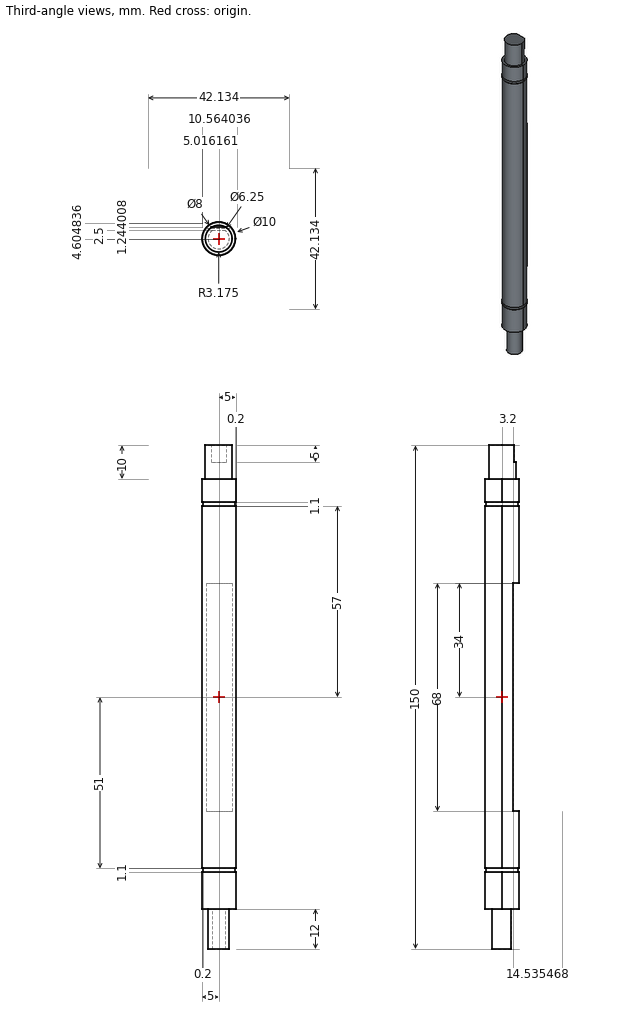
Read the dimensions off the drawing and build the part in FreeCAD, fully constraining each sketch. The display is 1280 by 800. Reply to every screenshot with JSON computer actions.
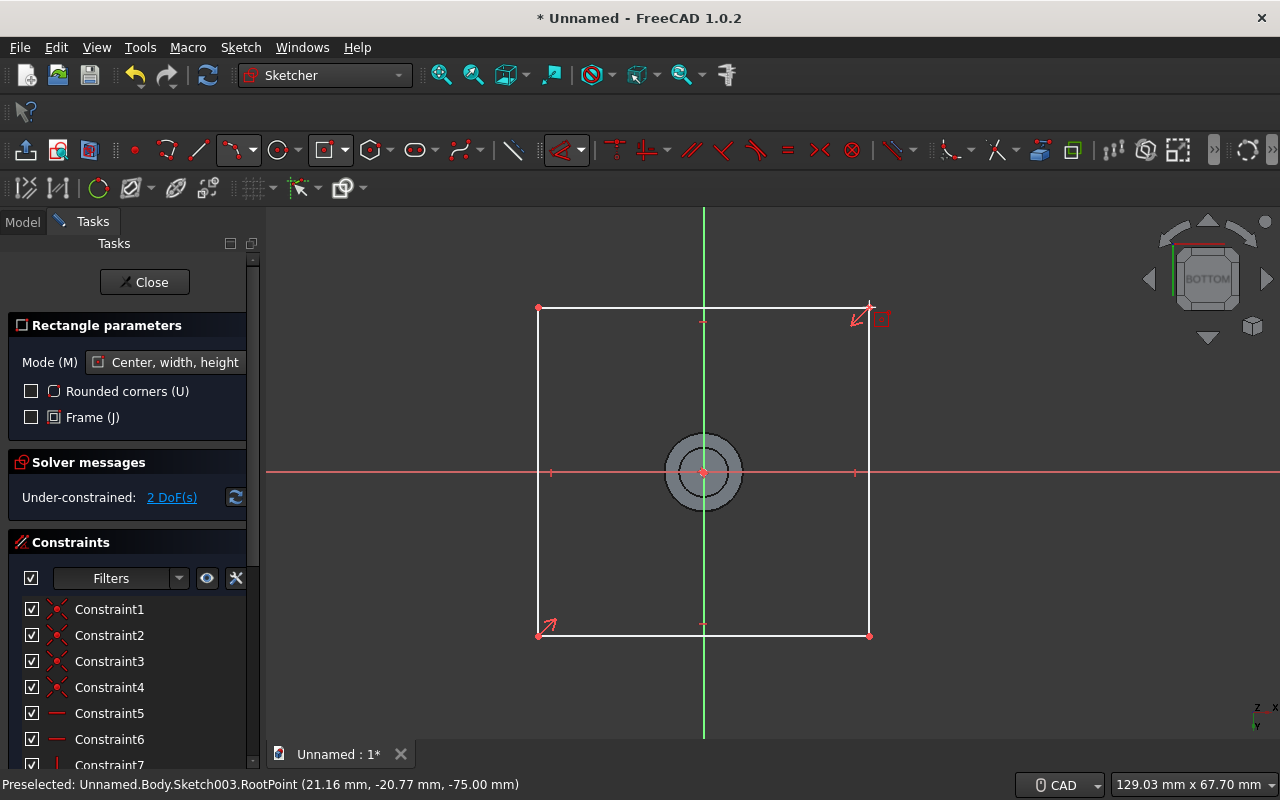
{"action": "left_click", "coordinate": [200, 150]}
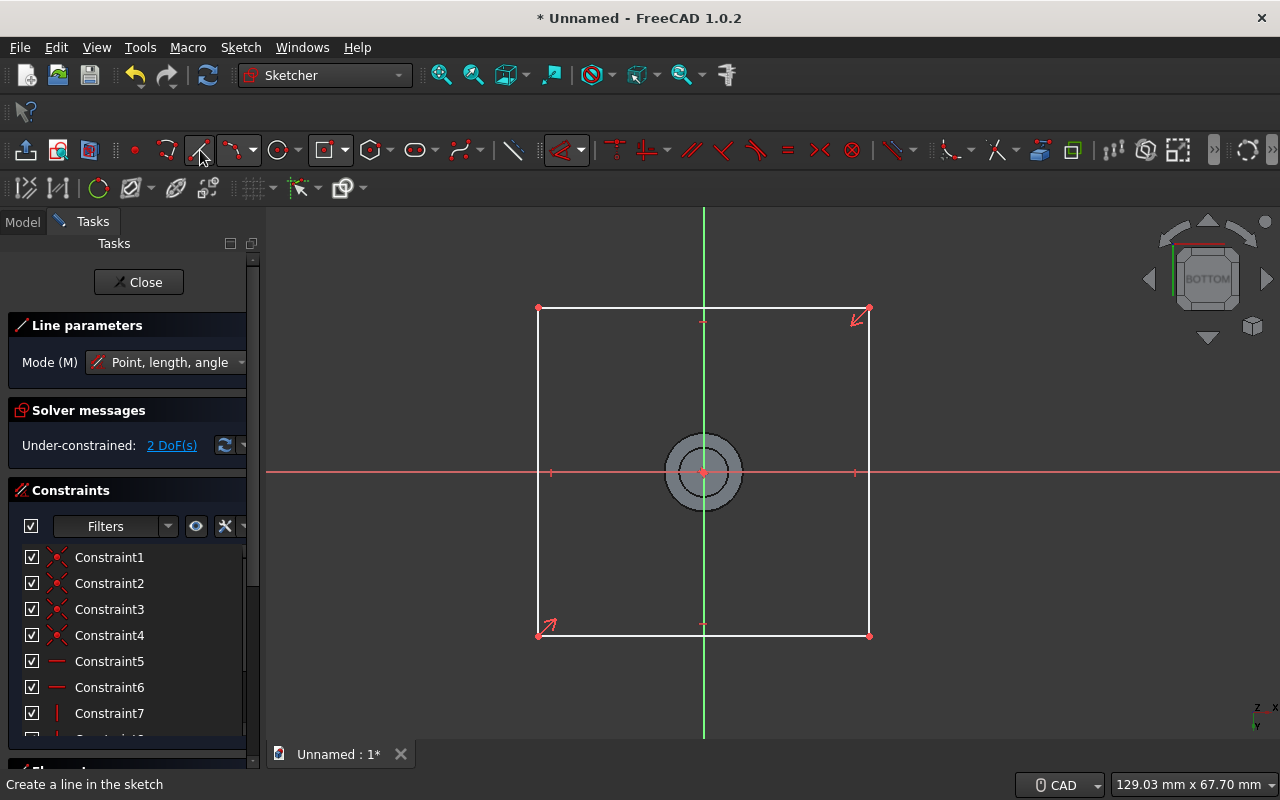
{"action": "left_click", "coordinate": [688, 492]}
{"action": "left_click", "coordinate": [719, 492]}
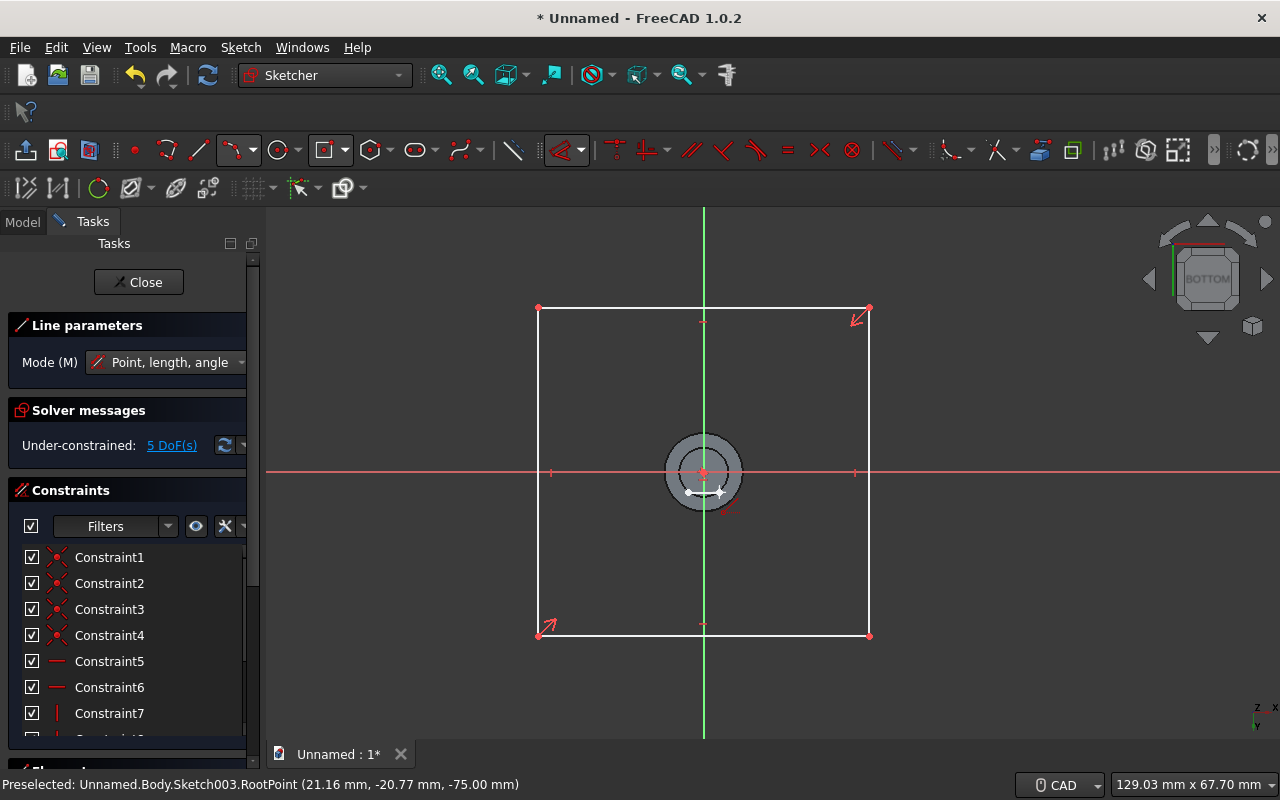
{"action": "left_click", "coordinate": [232, 150]}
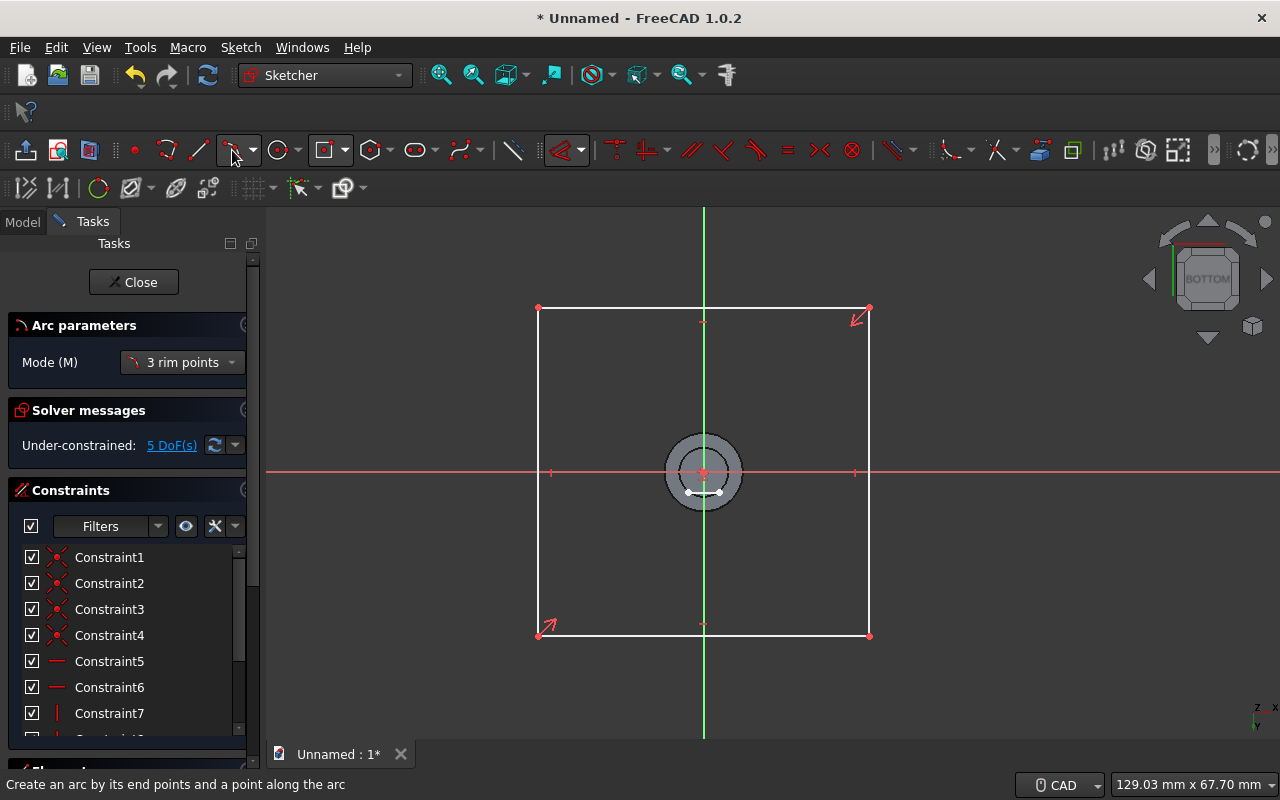
{"action": "left_click", "coordinate": [719, 493]}
{"action": "left_click", "coordinate": [688, 493]}
{"action": "left_click", "coordinate": [683, 459]}
{"action": "key", "text": "Escape"}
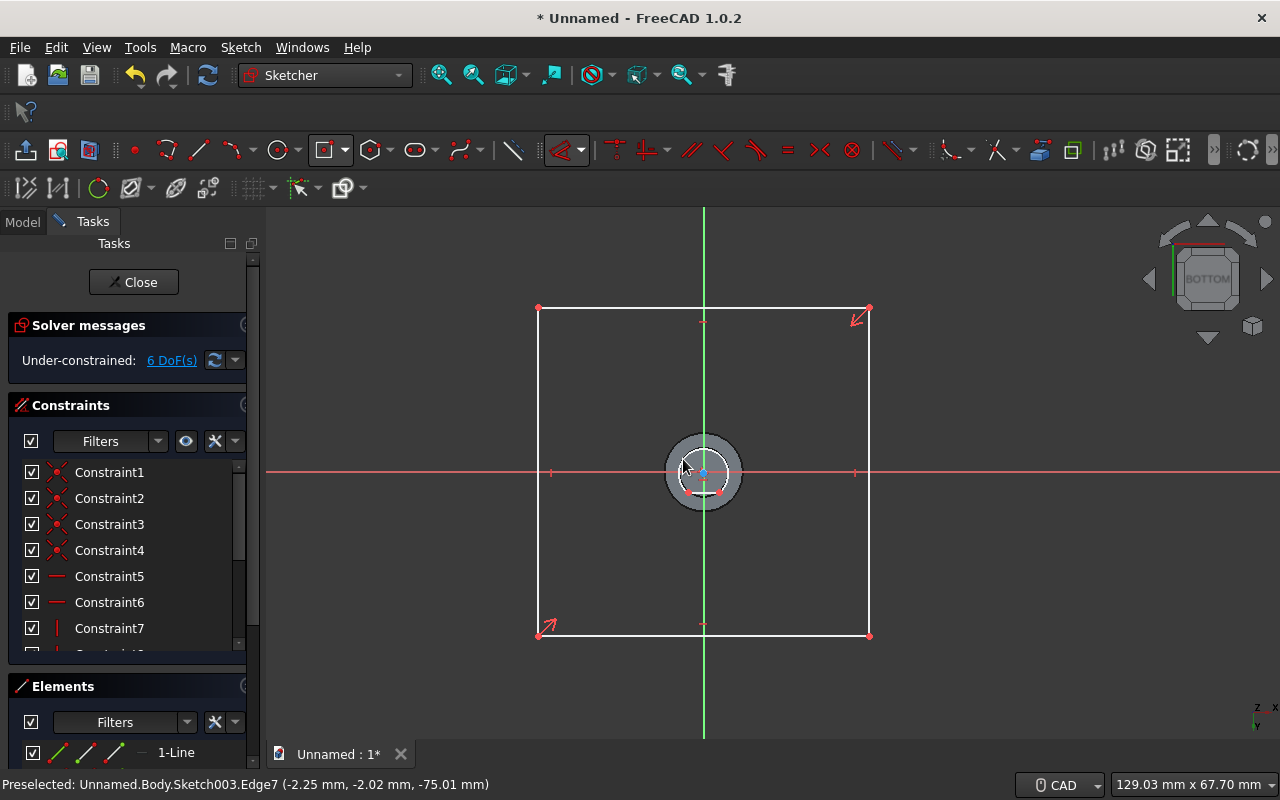
{"action": "scroll", "coordinate": [704, 473], "scroll_direction": "up", "scroll_amount": 3}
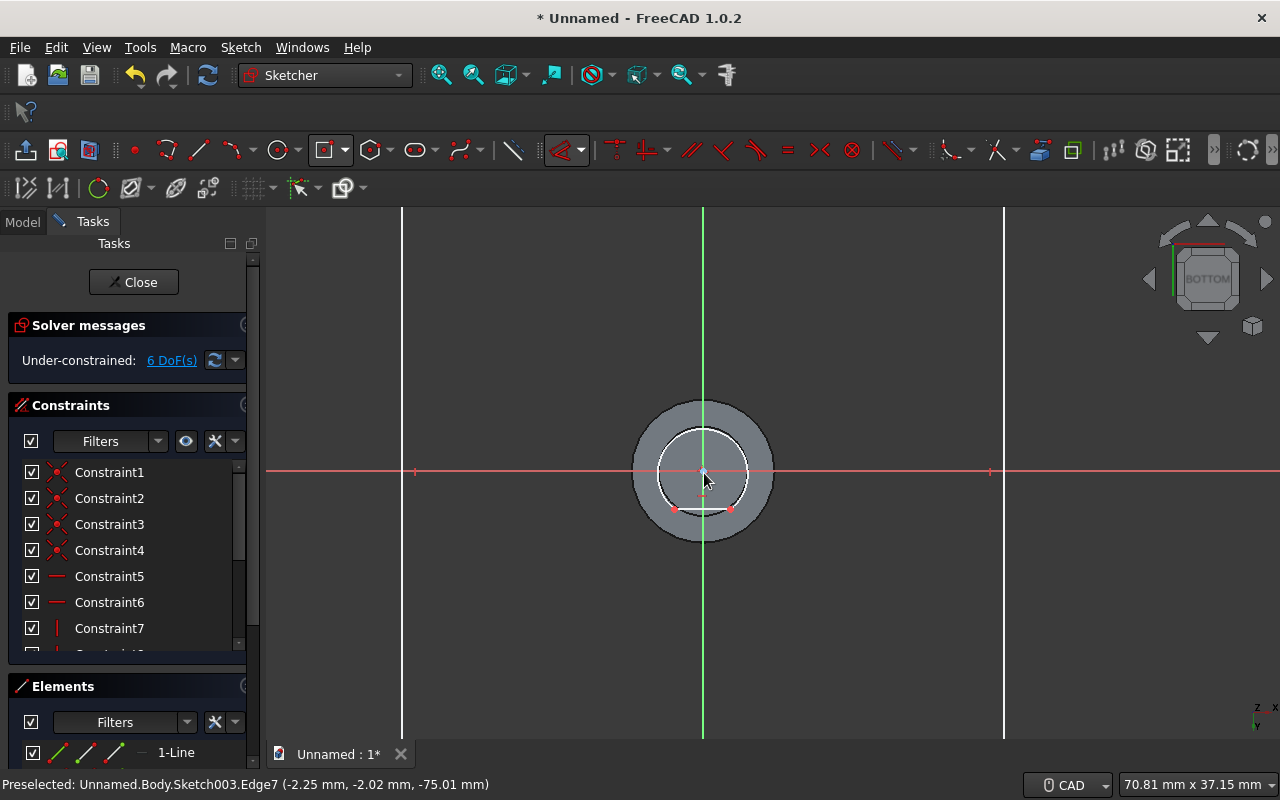
{"action": "left_click_drag", "start_coordinate": [693, 461], "coordinate": [713, 484]}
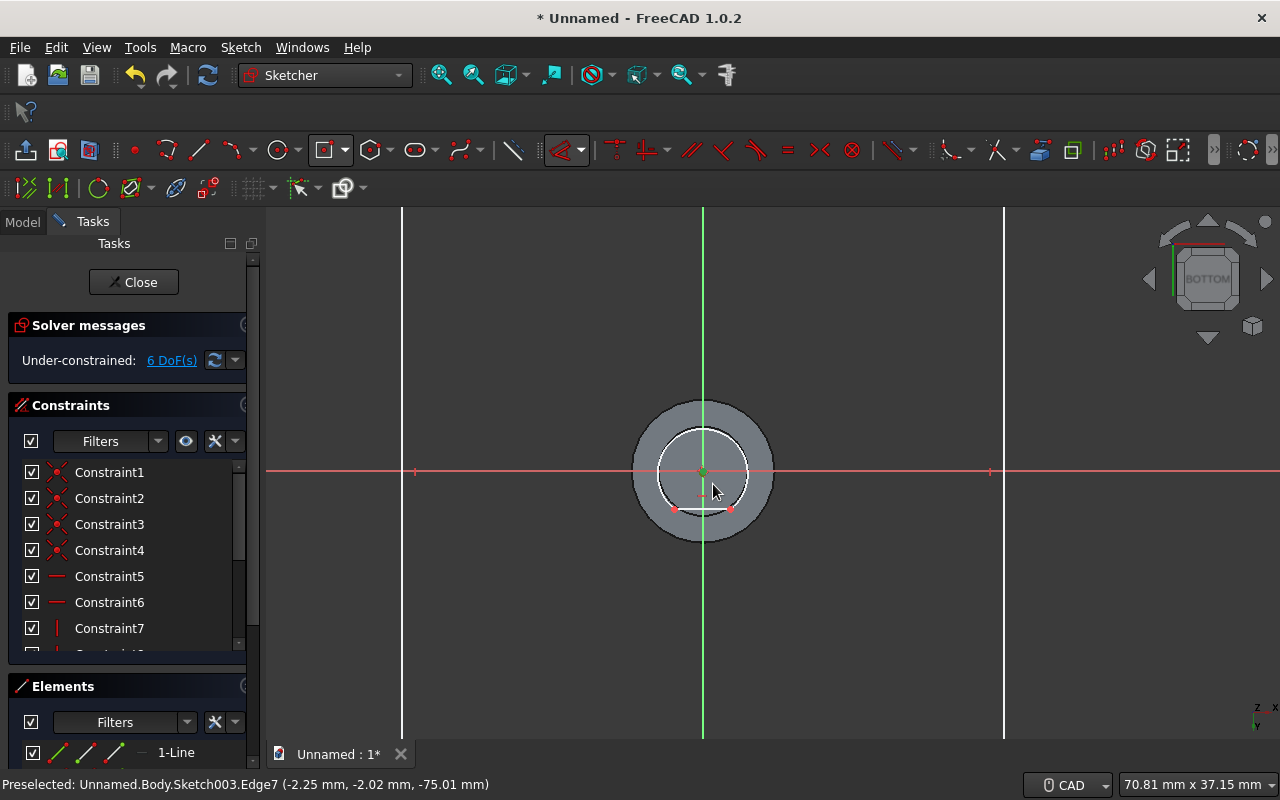
{"action": "left_click", "coordinate": [616, 150]}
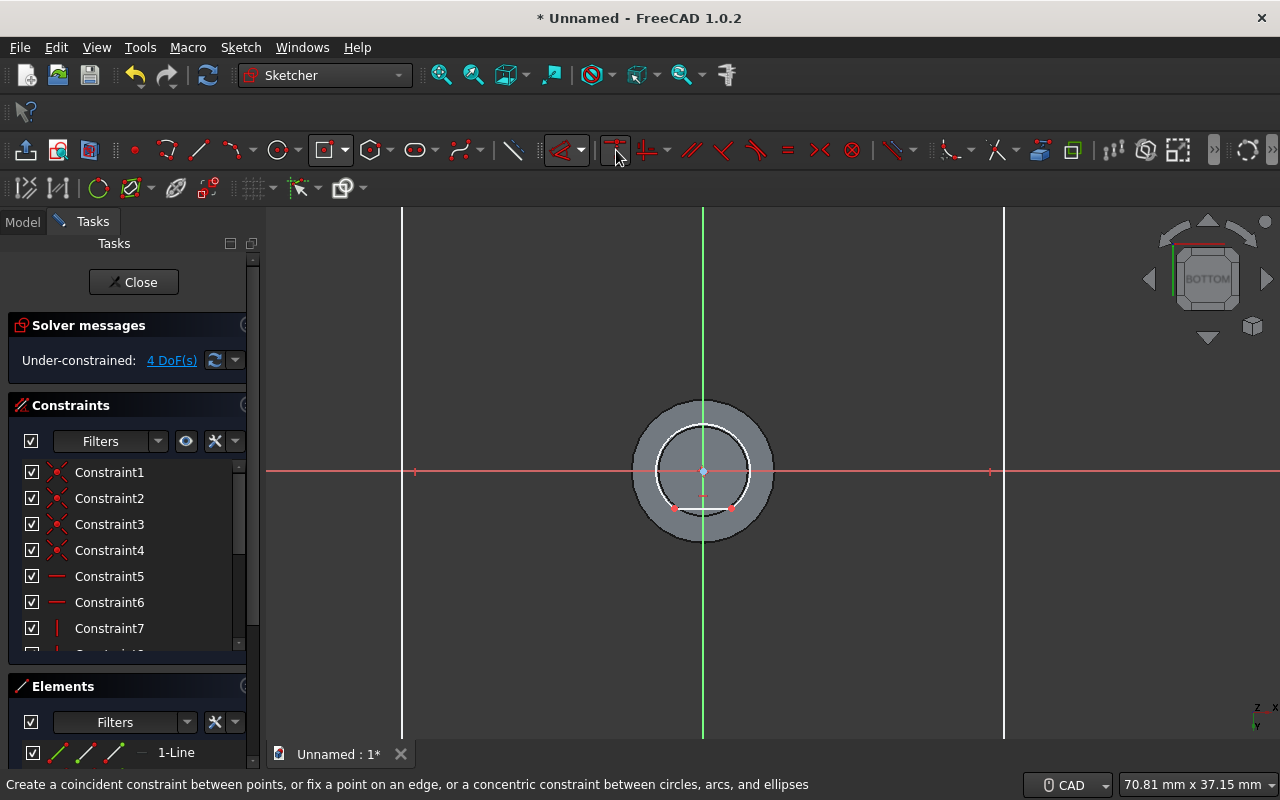
{"action": "left_click", "coordinate": [743, 446]}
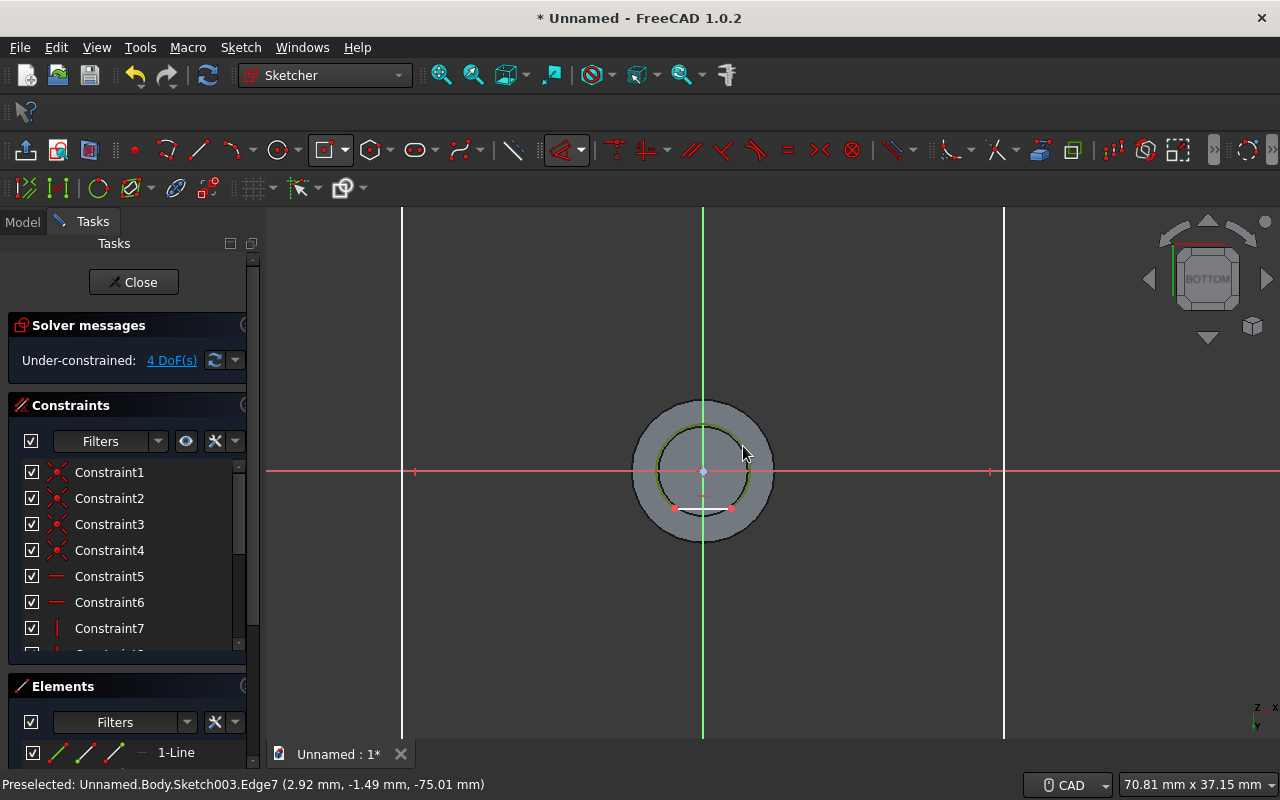
{"action": "key", "text": "k r"}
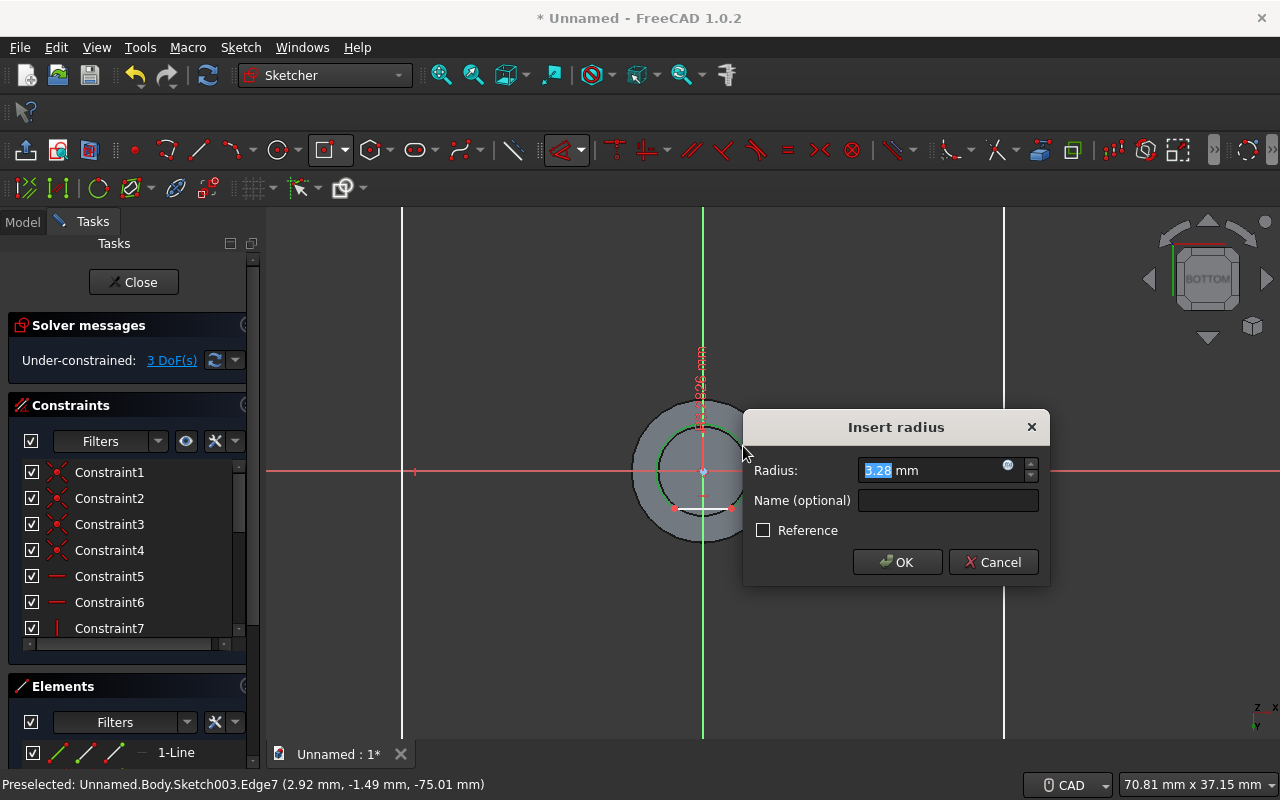
{"action": "type", "text": "3.175"}
{"action": "key", "text": "Return"}